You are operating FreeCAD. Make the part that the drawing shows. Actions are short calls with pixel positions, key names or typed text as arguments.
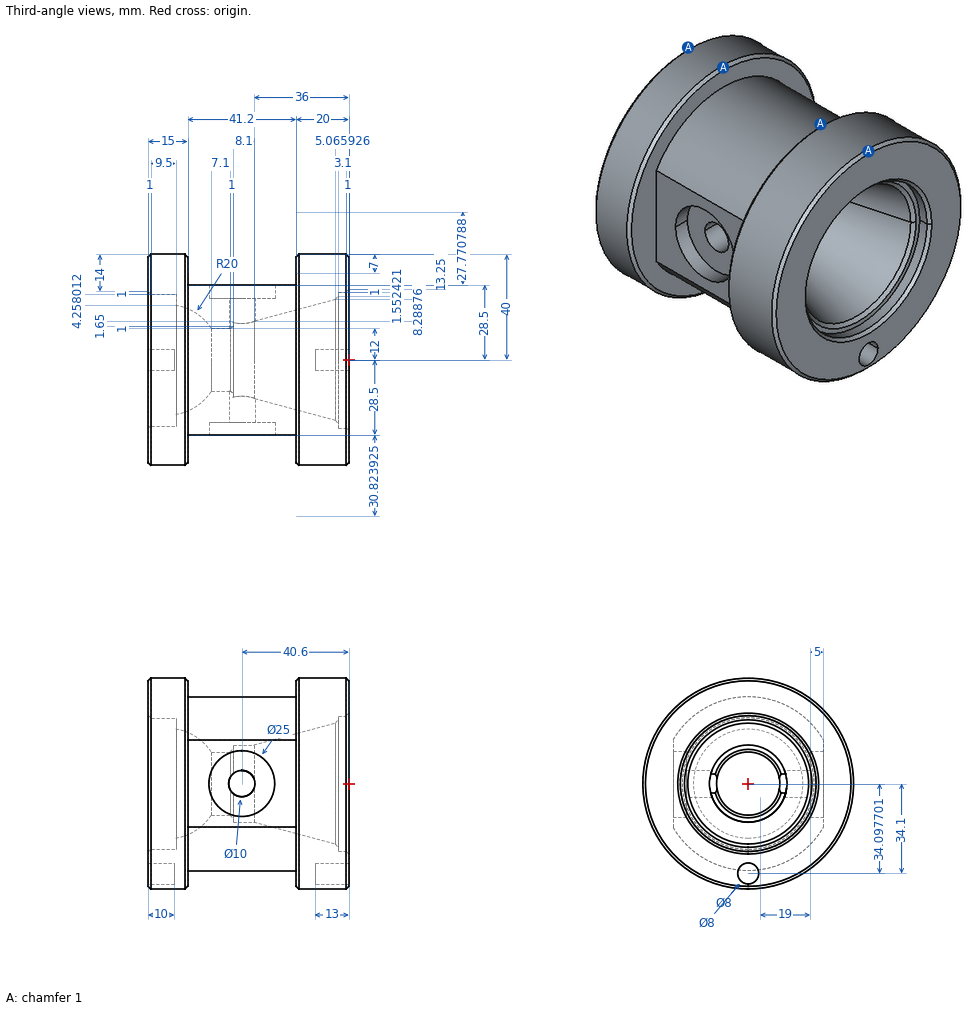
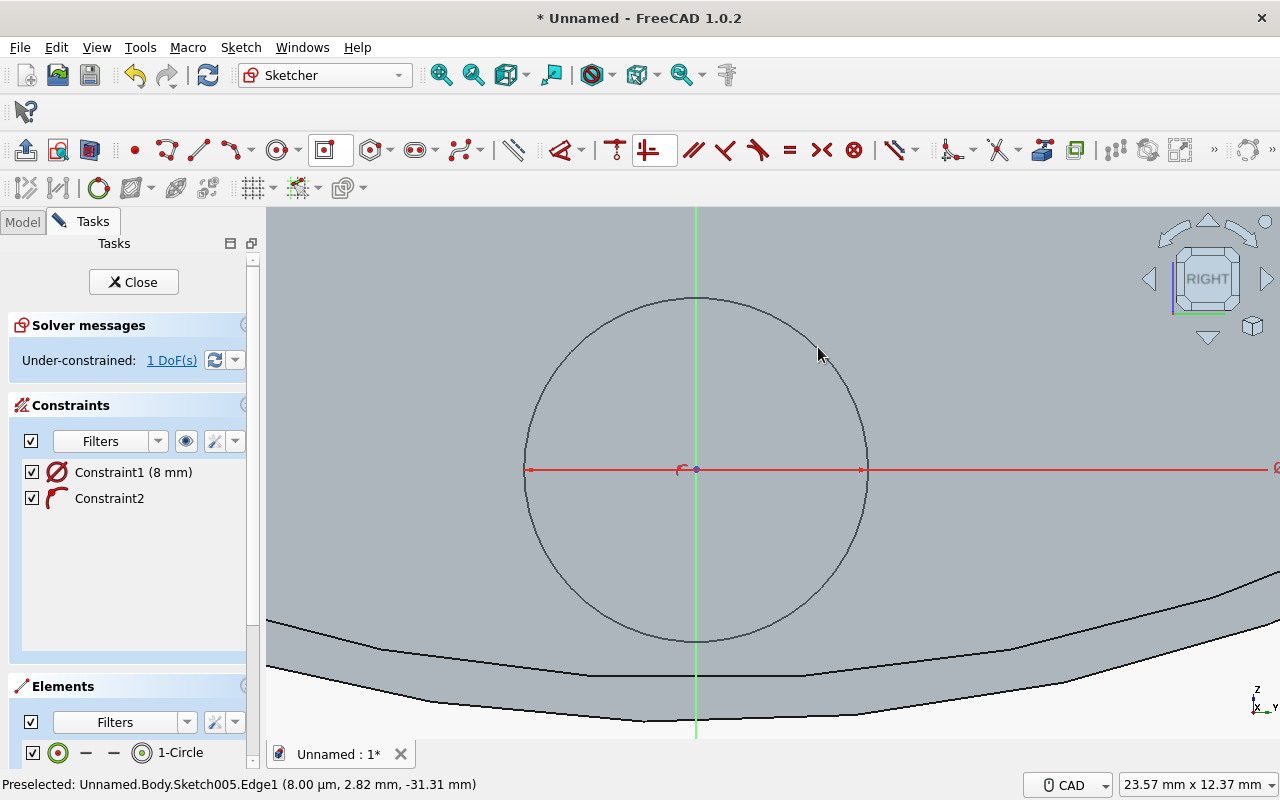
click(560, 150)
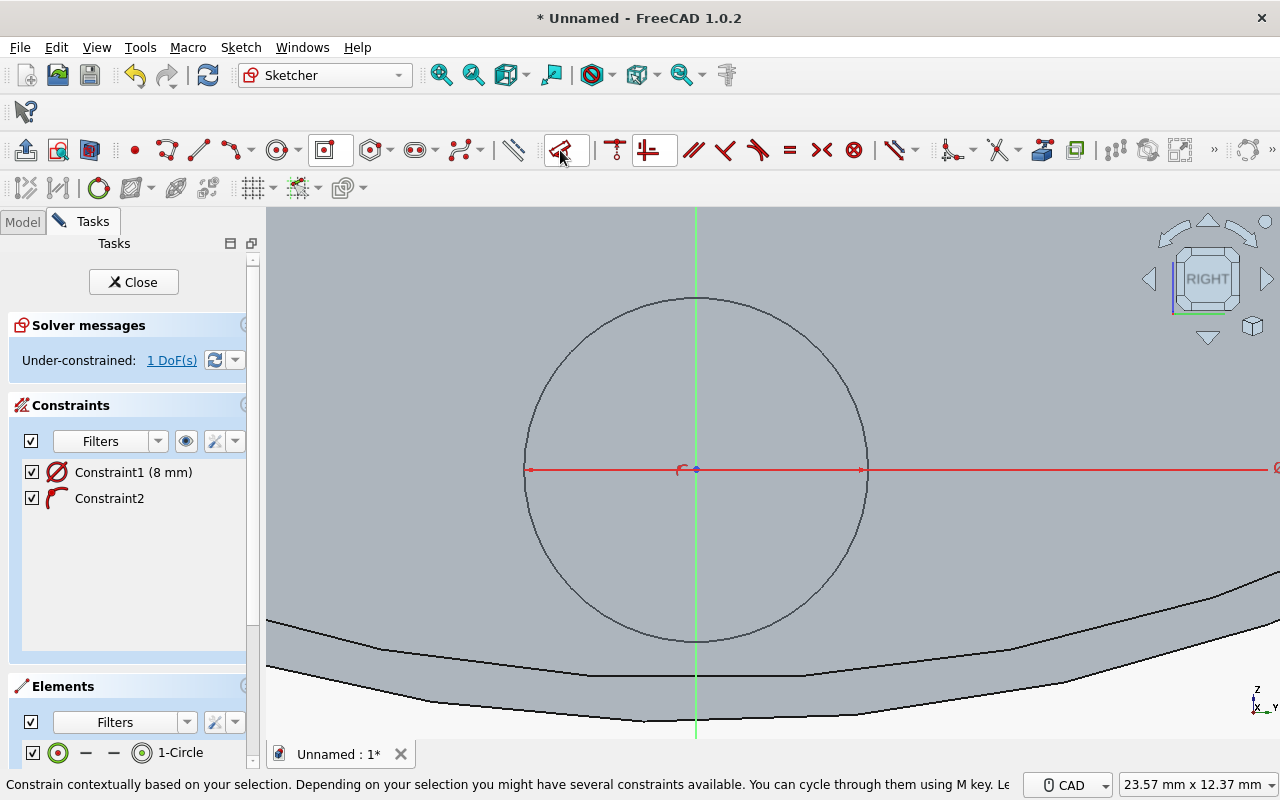
click(696, 470)
click(730, 352)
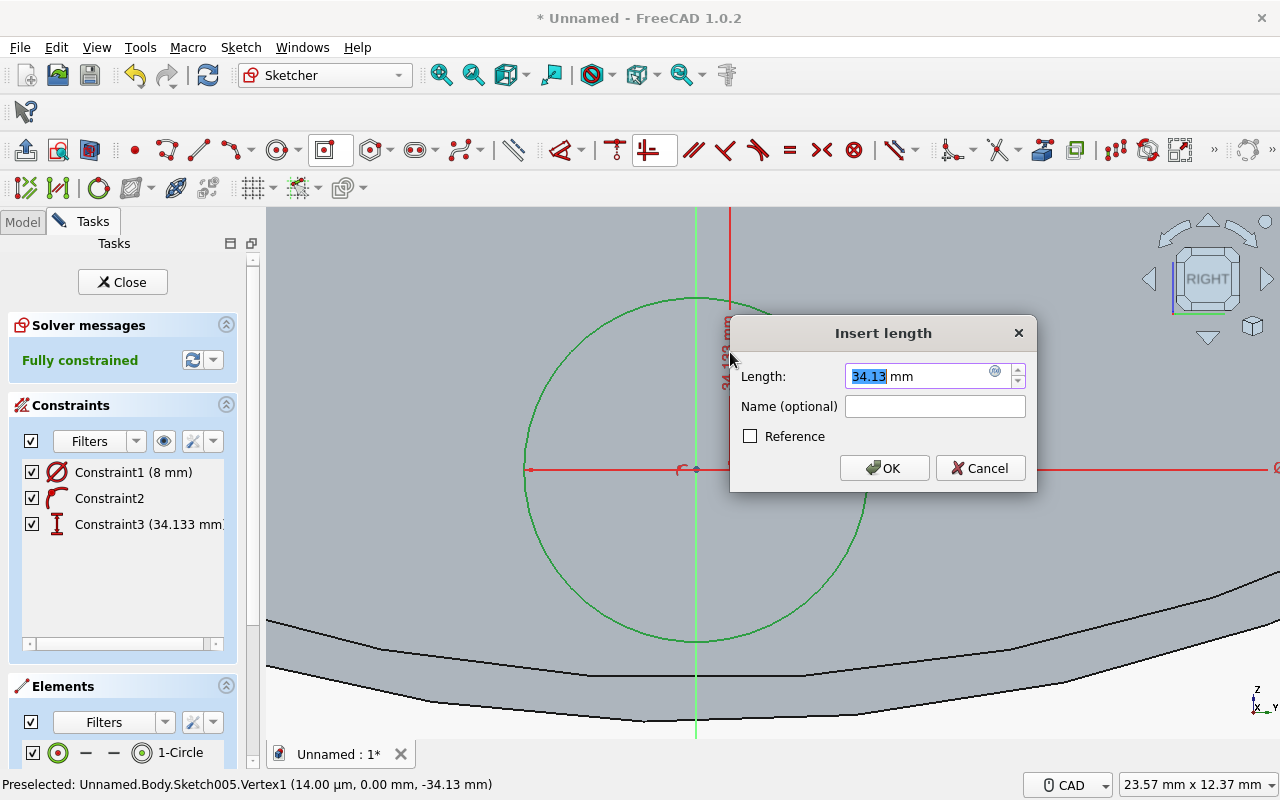
text(34.1)
key(Return)
key(Escape)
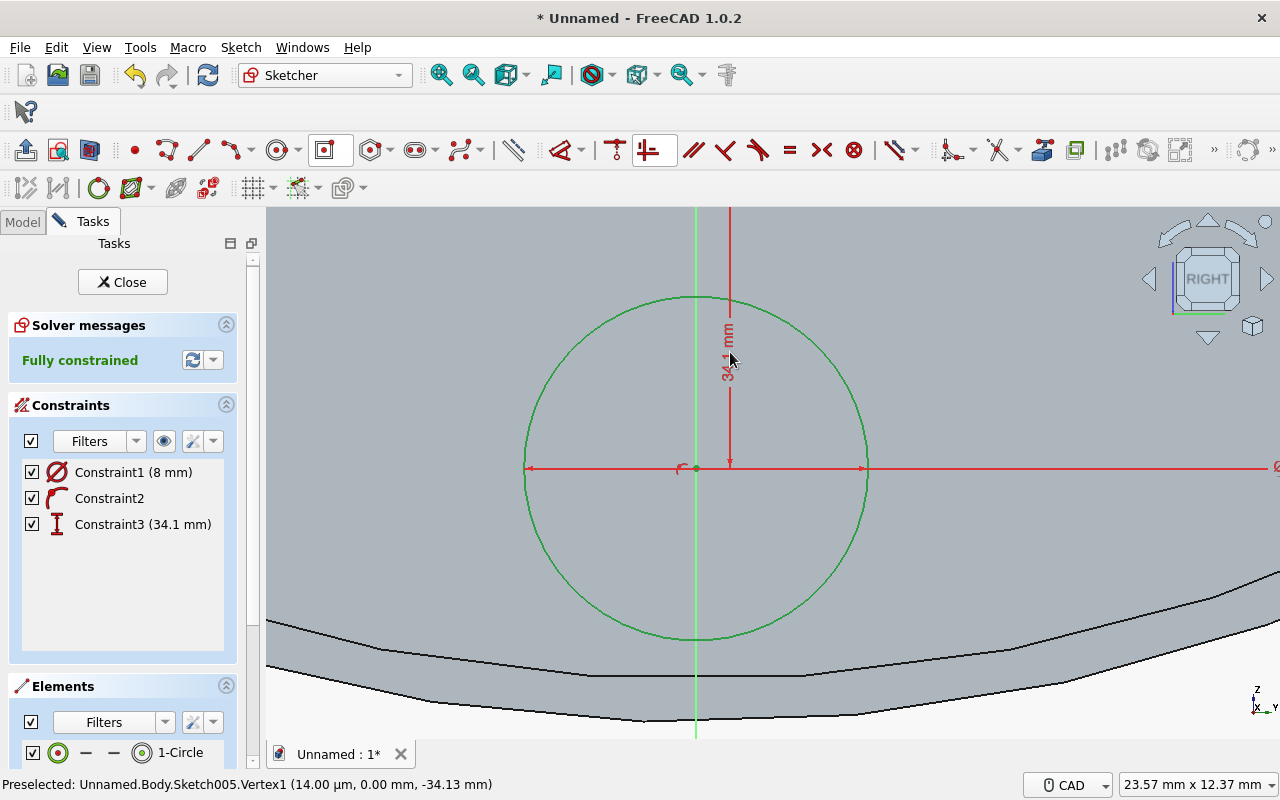
click(123, 282)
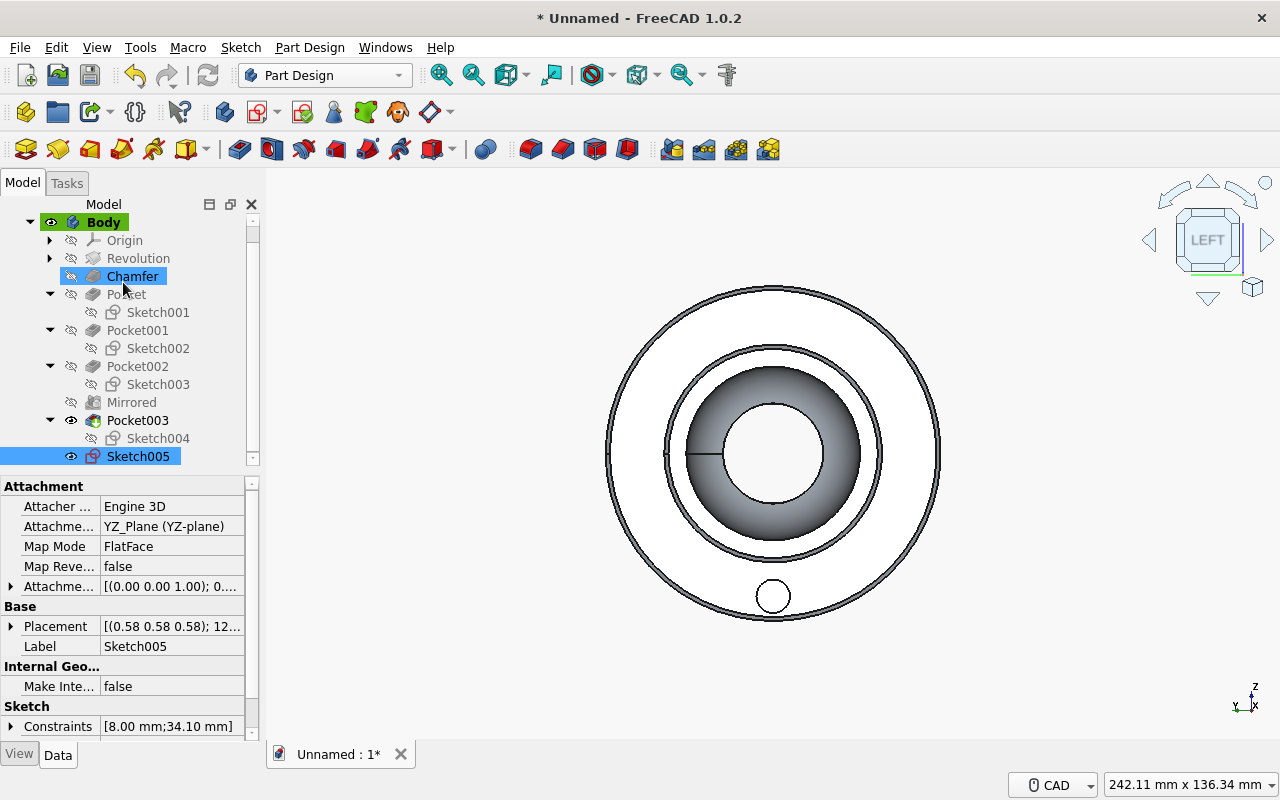
click(240, 150)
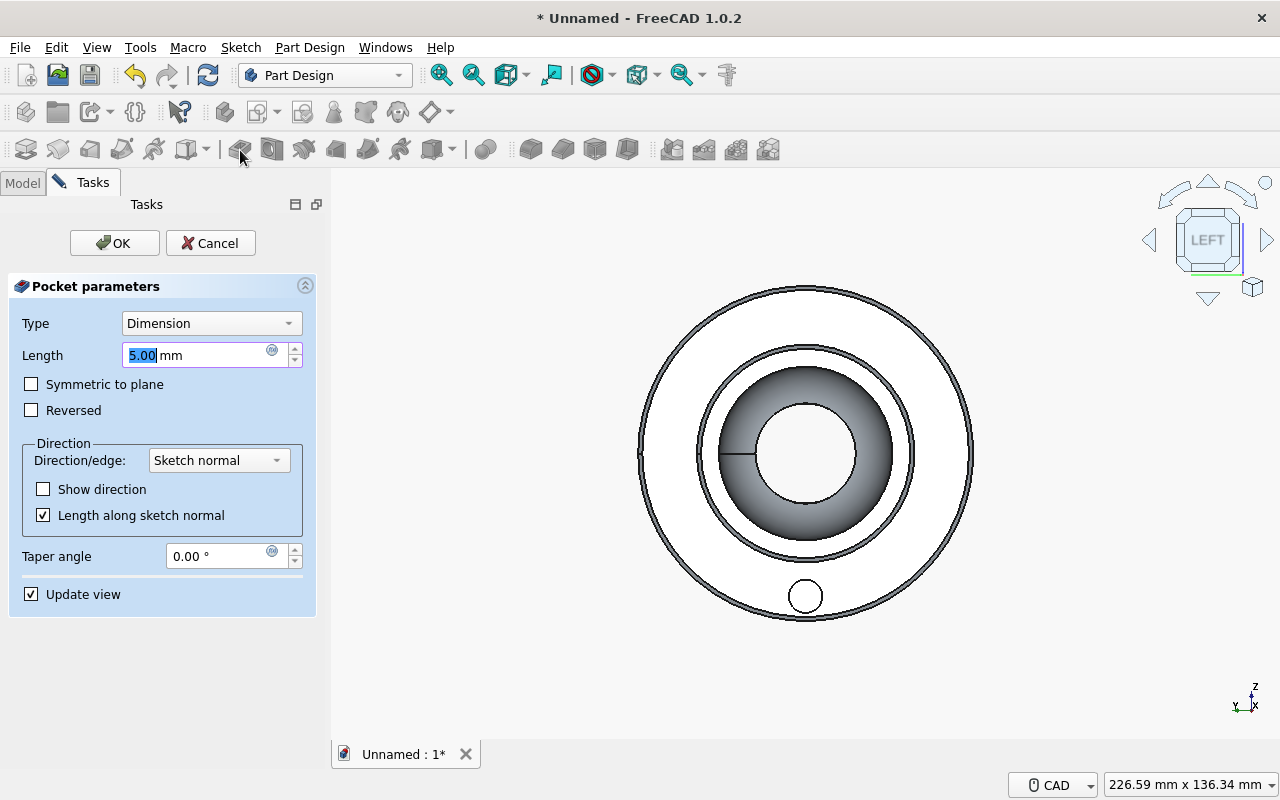
text(13)
key(Tab)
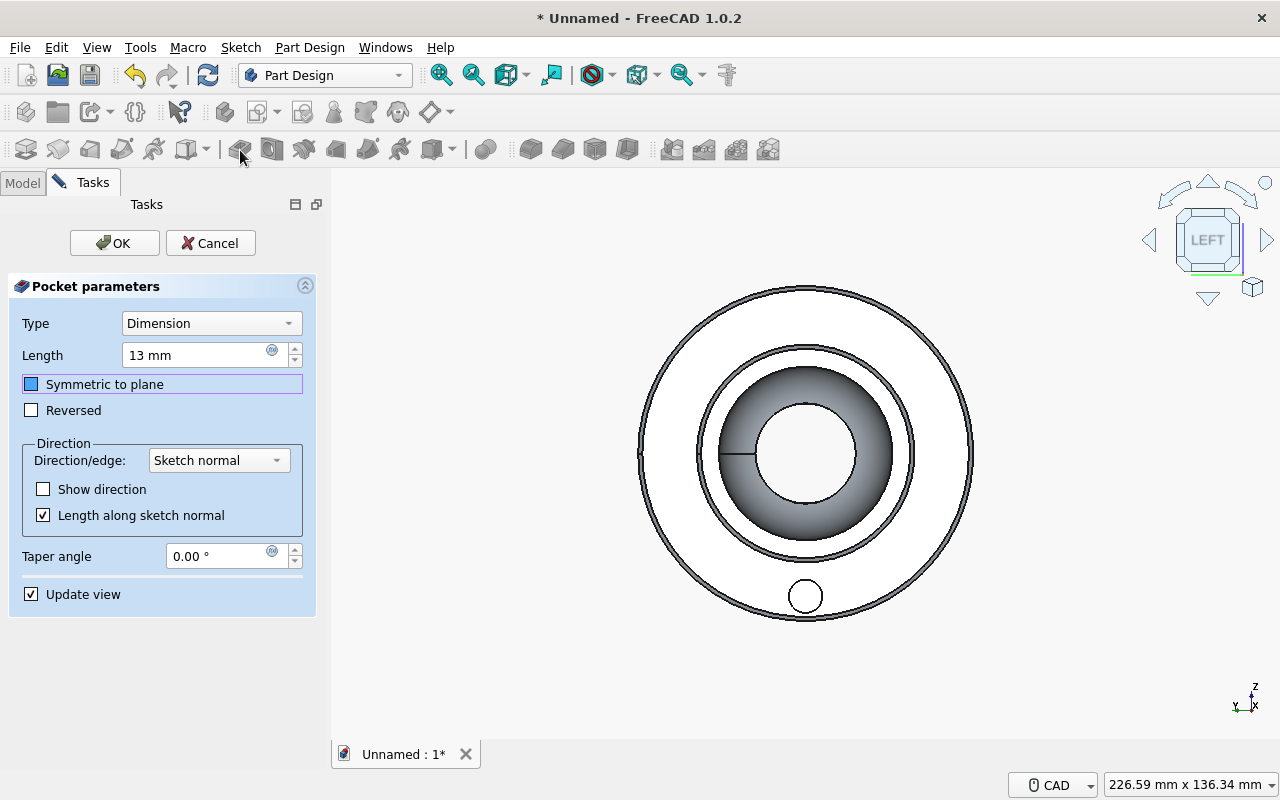
click(115, 243)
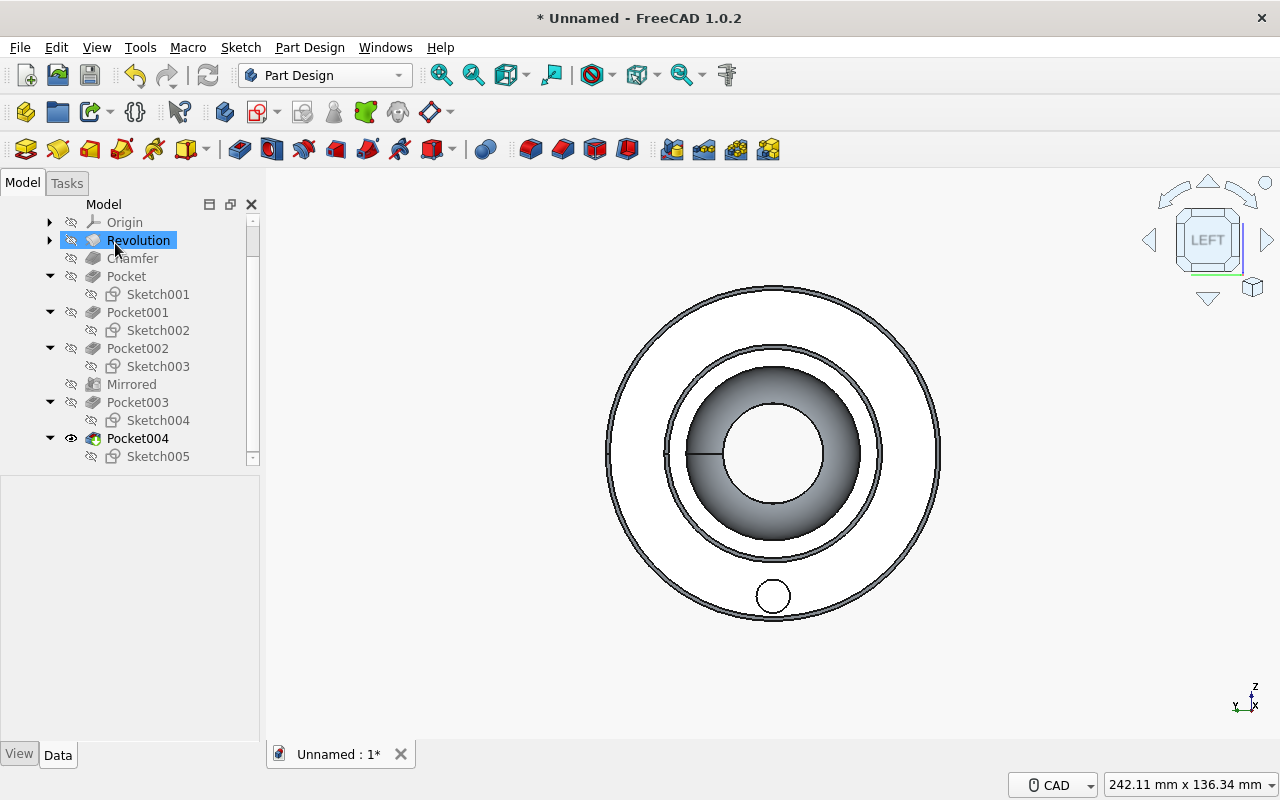
key(0)